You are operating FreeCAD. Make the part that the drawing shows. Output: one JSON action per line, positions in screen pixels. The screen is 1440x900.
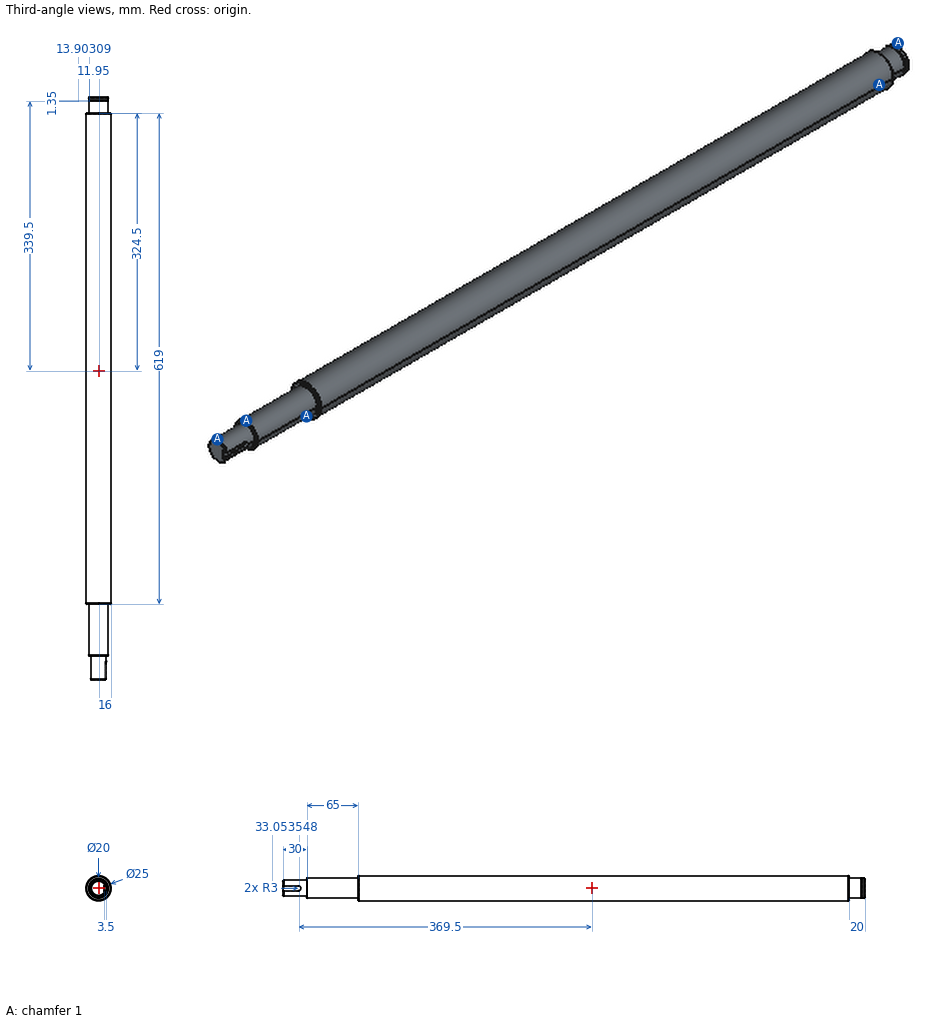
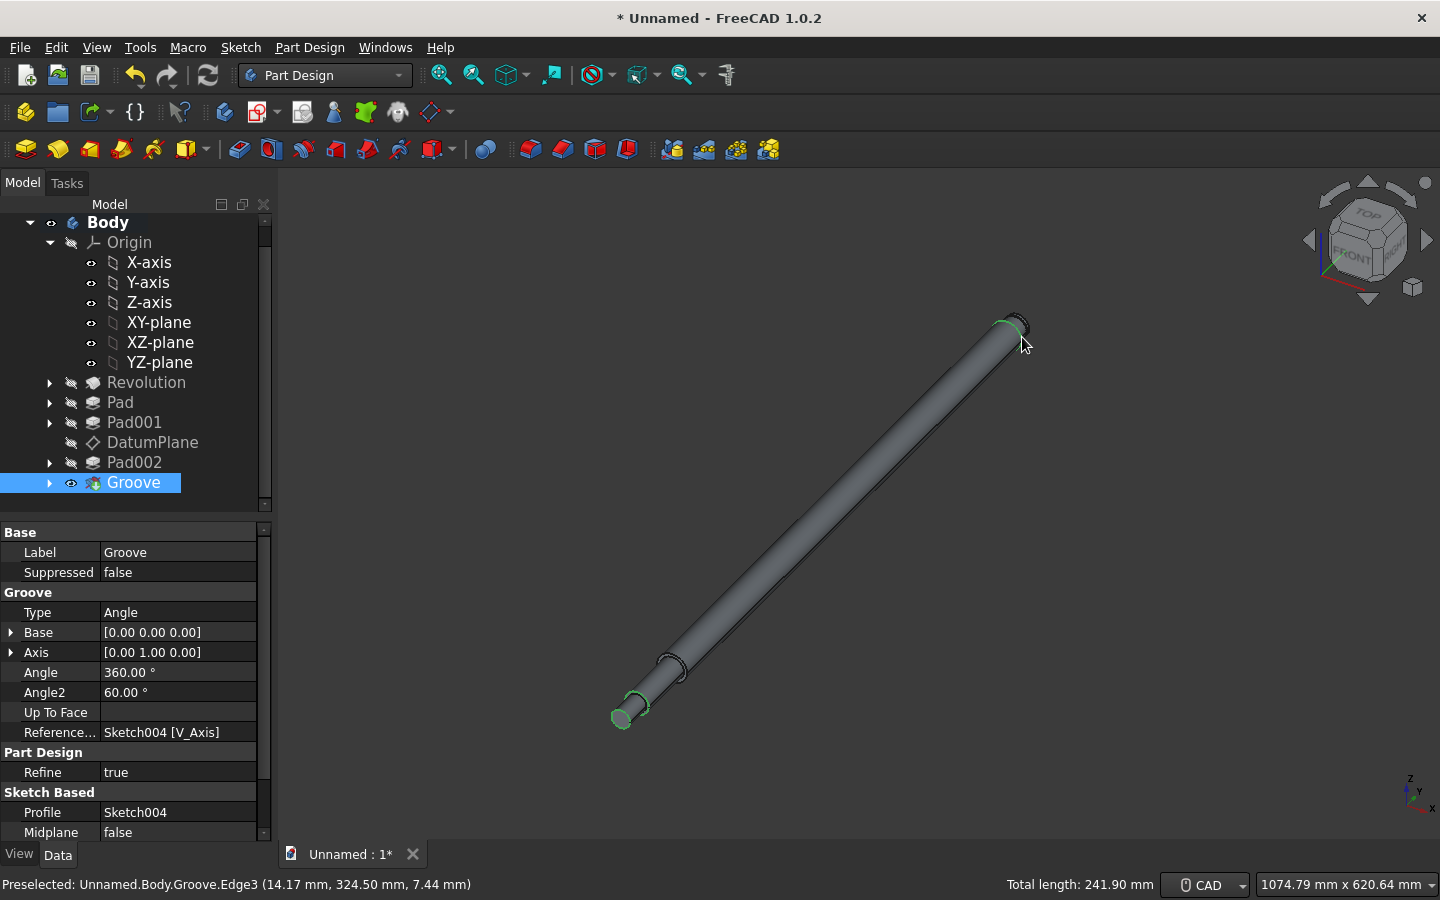
{"action": "left_click", "coordinate": [660, 655], "text": "ctrl"}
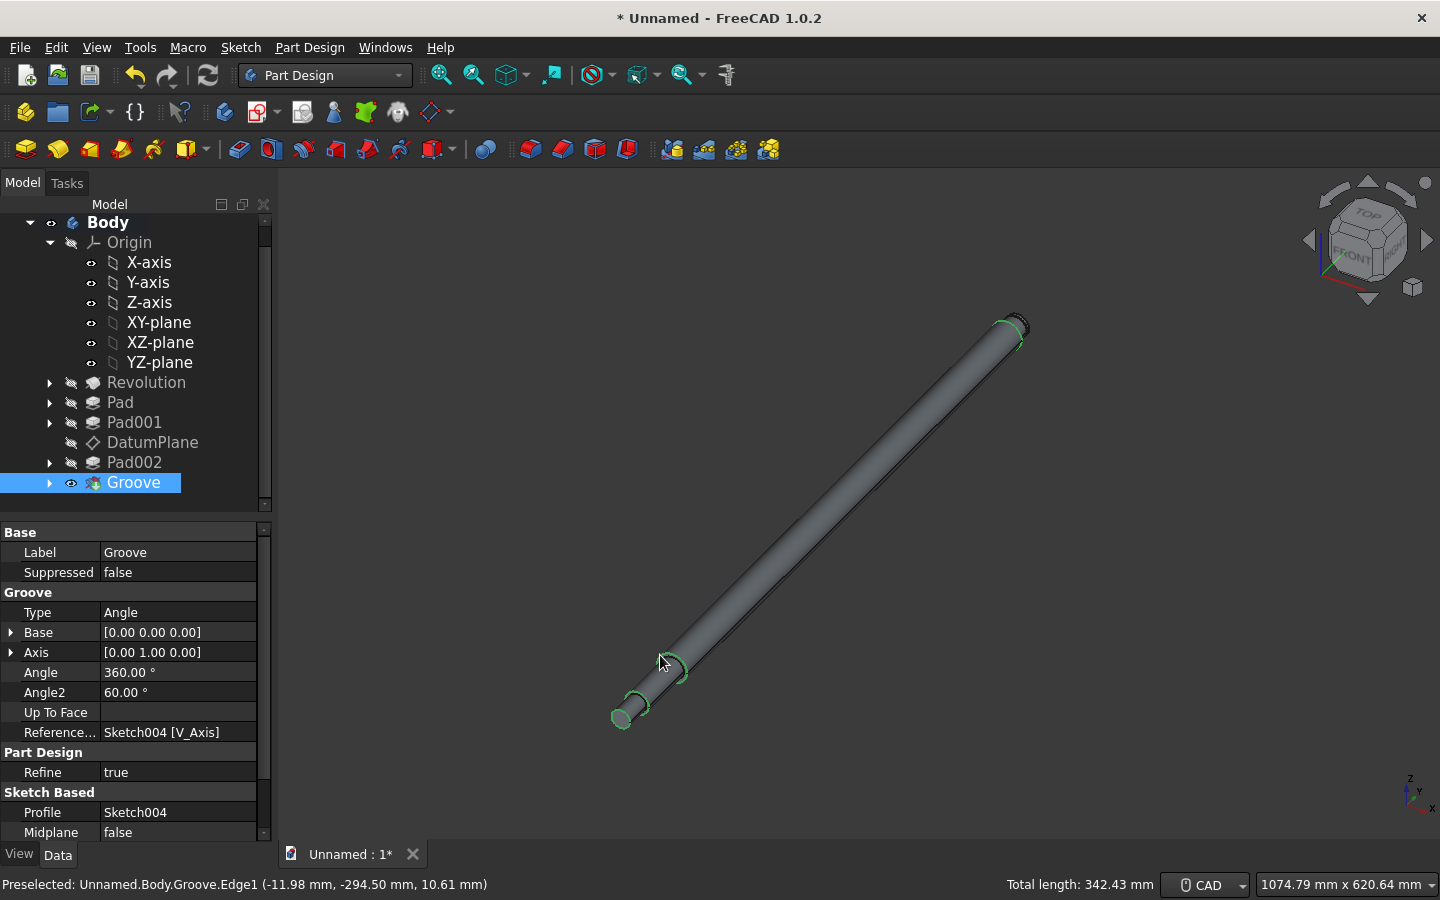
{"action": "key", "text": "0"}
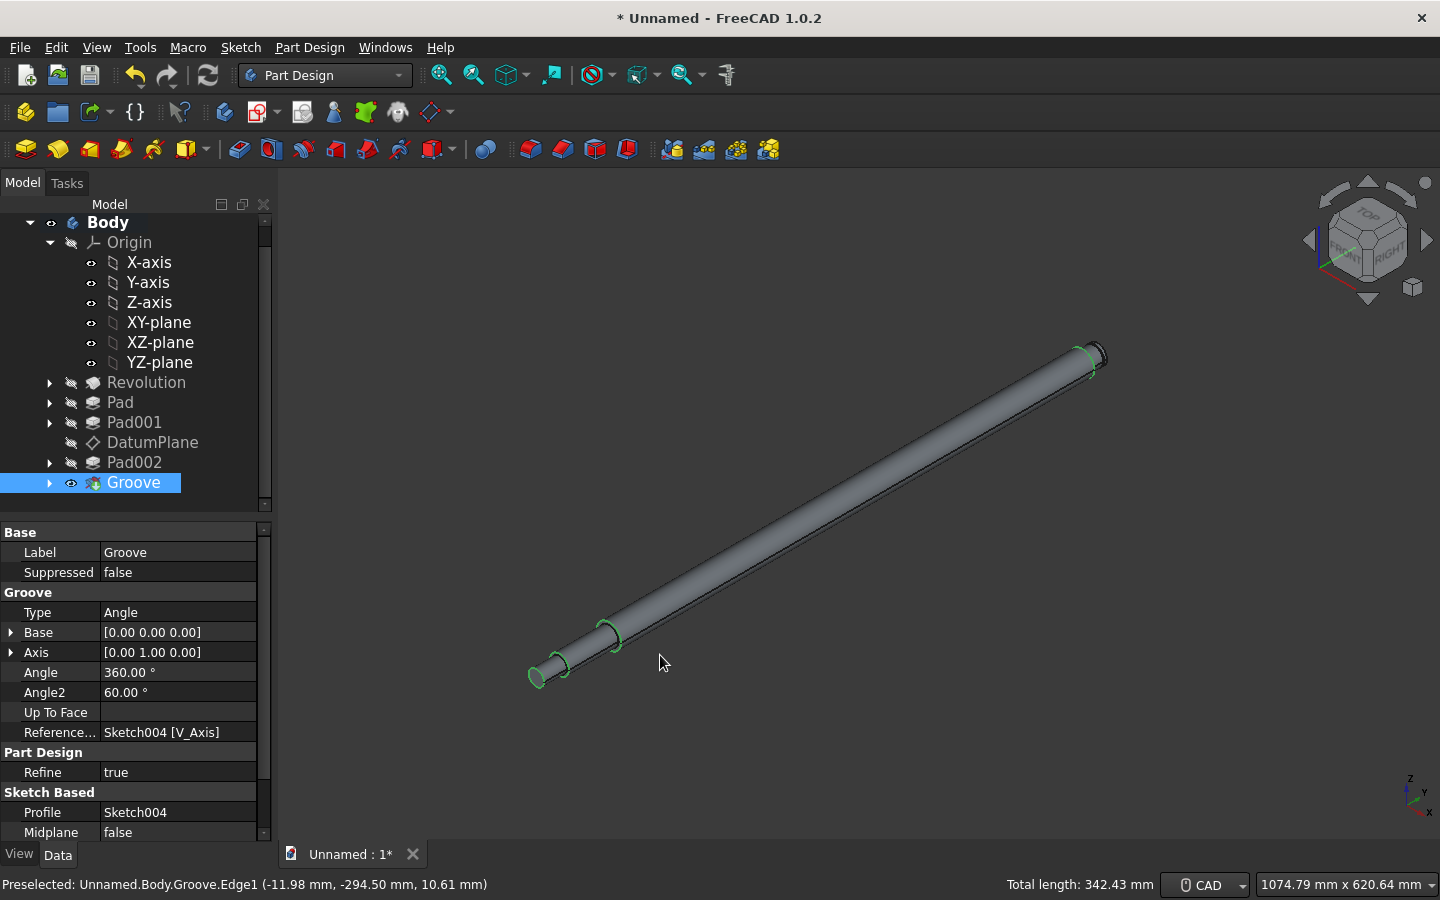
{"action": "key", "text": "2"}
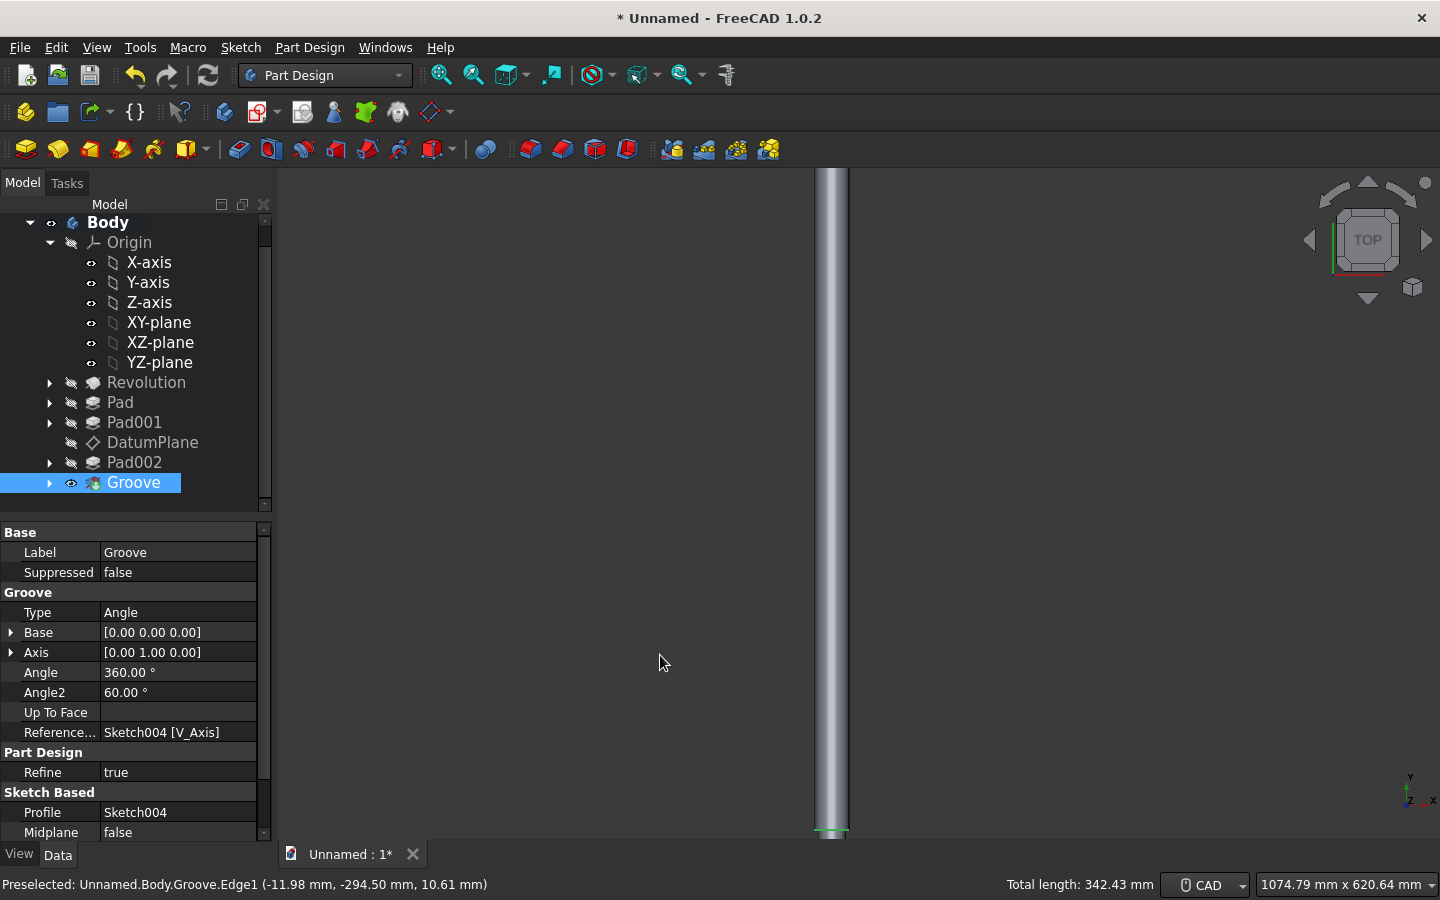
{"action": "left_click", "coordinate": [442, 76]}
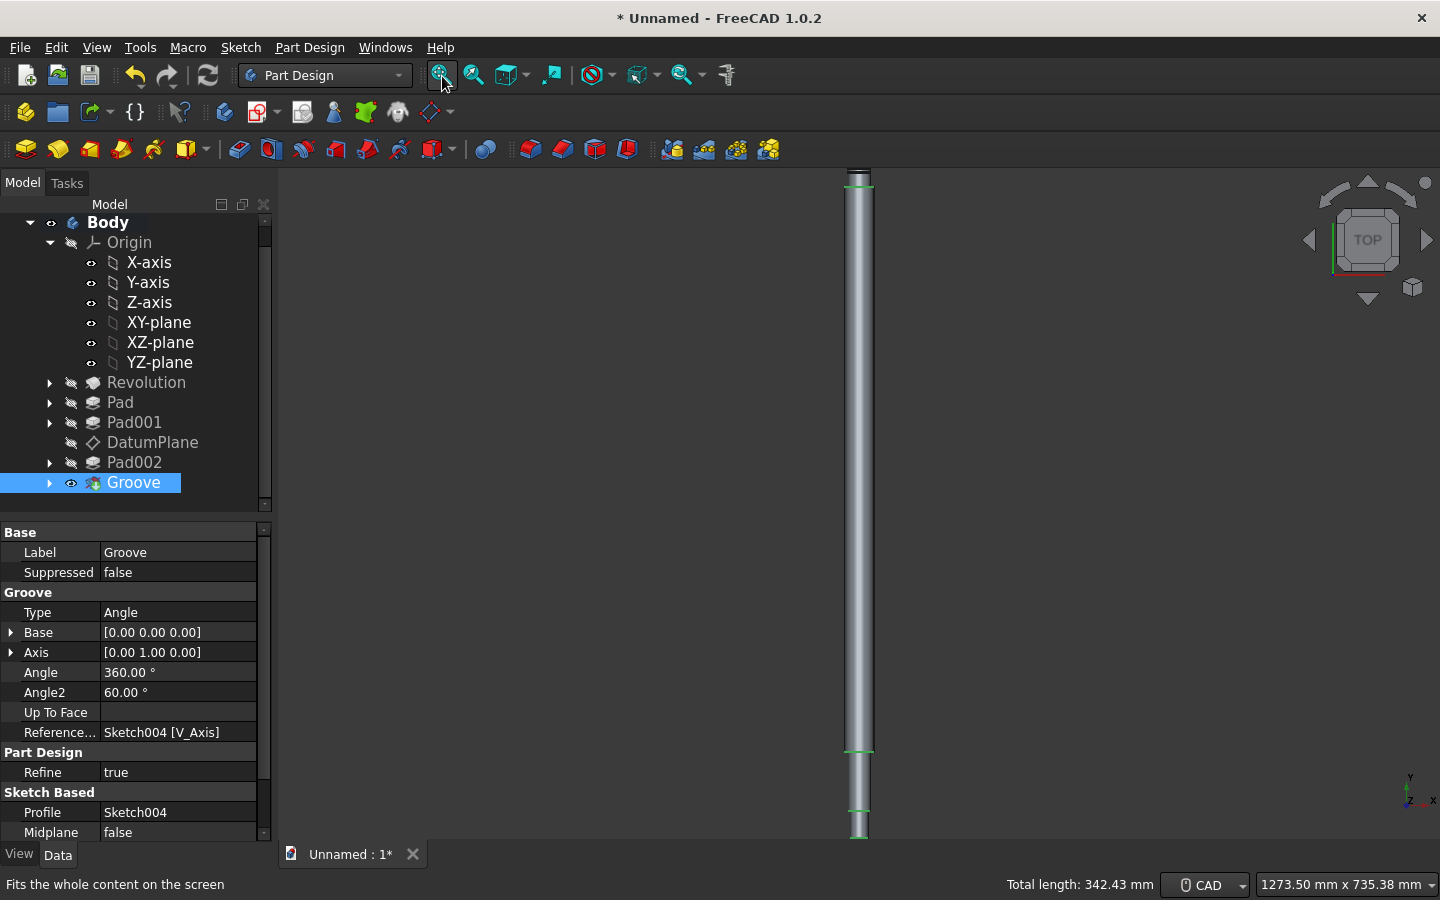
{"action": "key", "text": "1"}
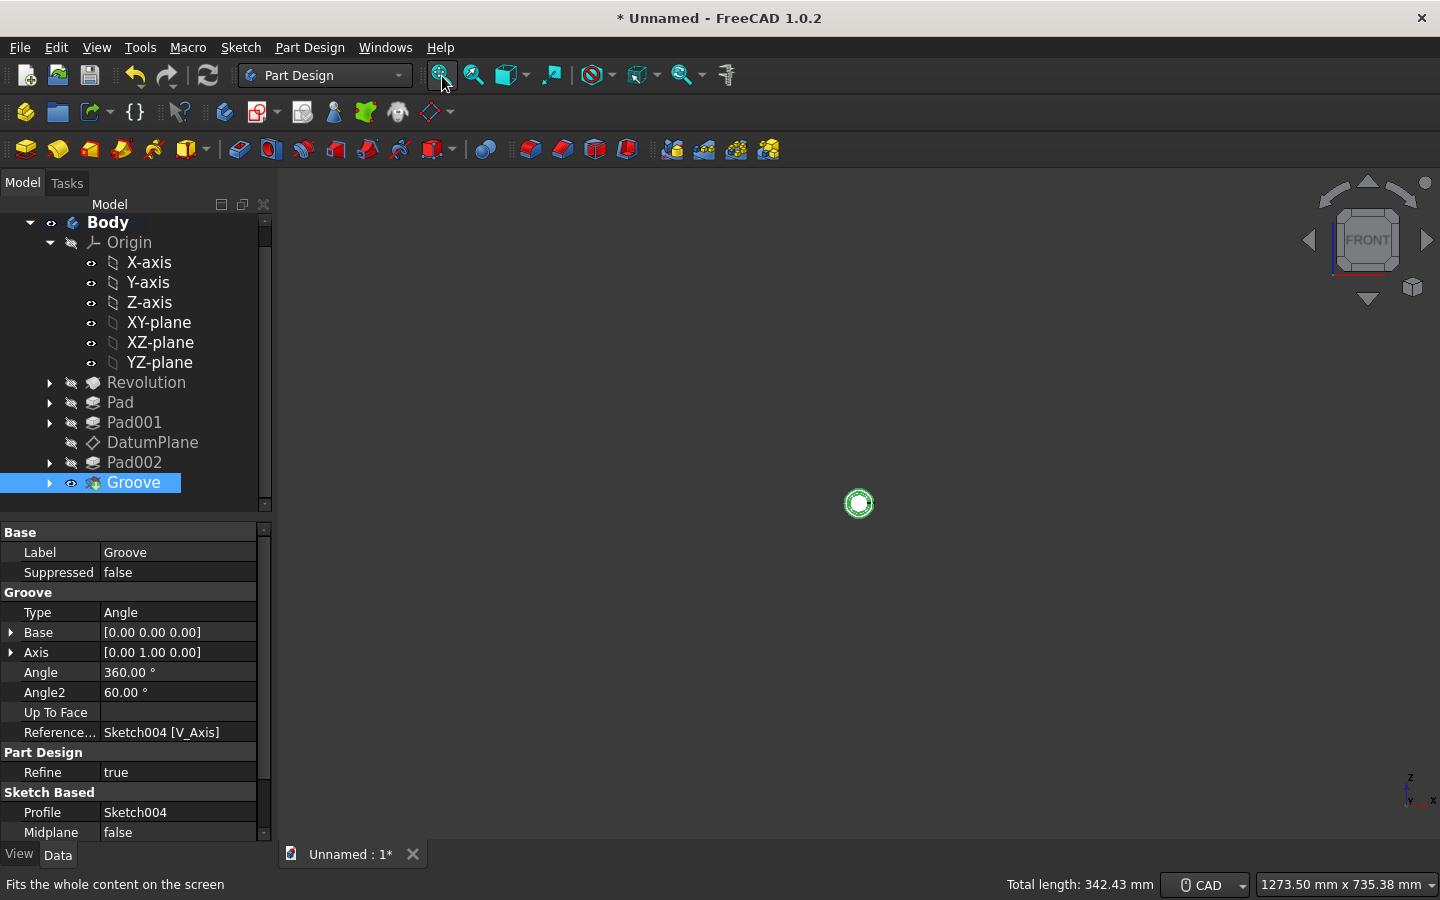
{"action": "left_click", "coordinate": [442, 76]}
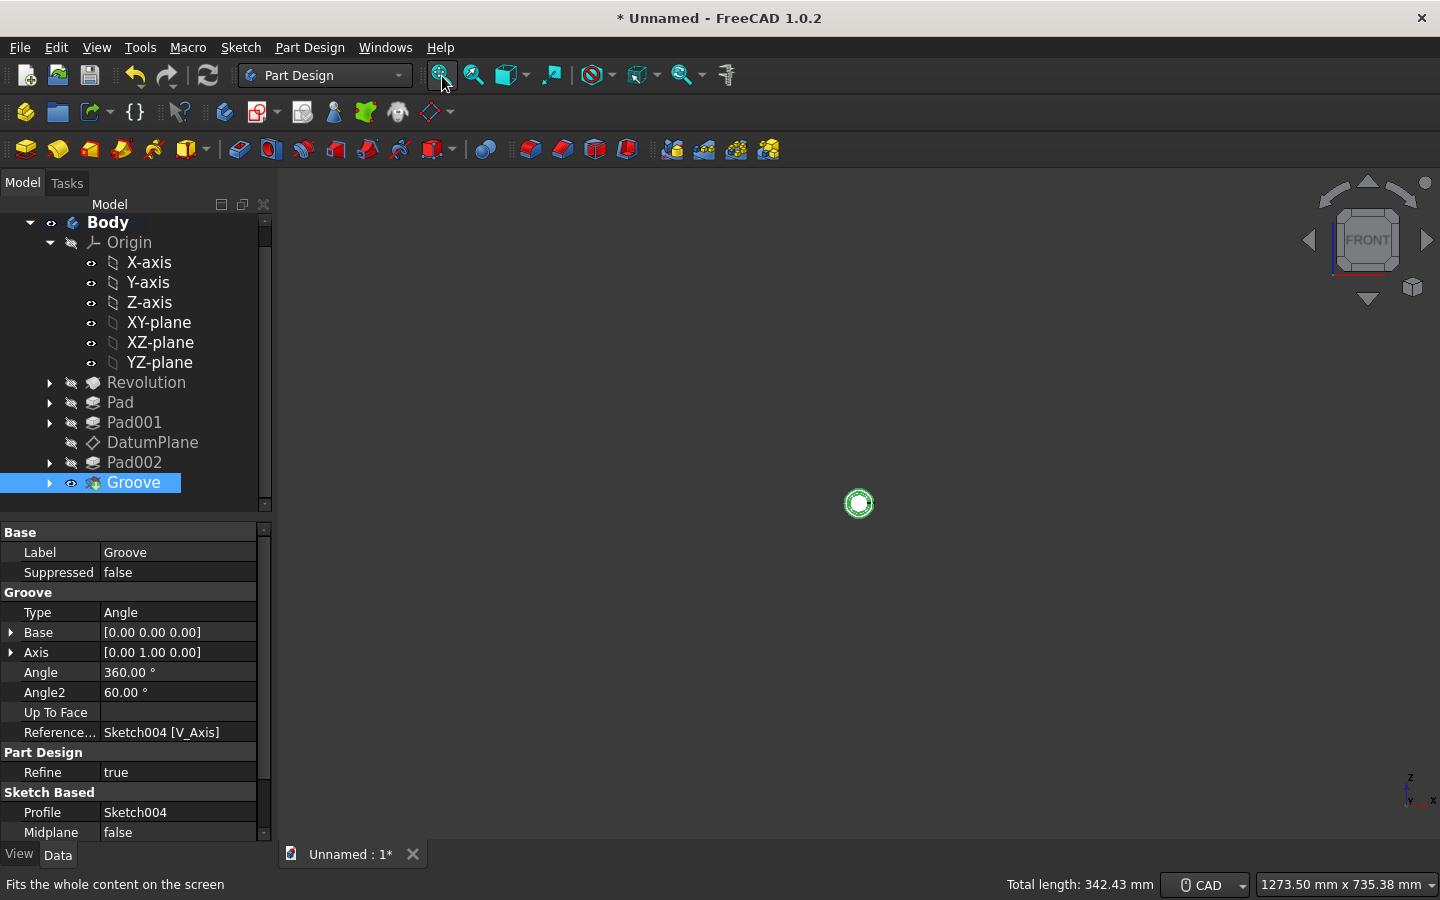
{"action": "key", "text": "3"}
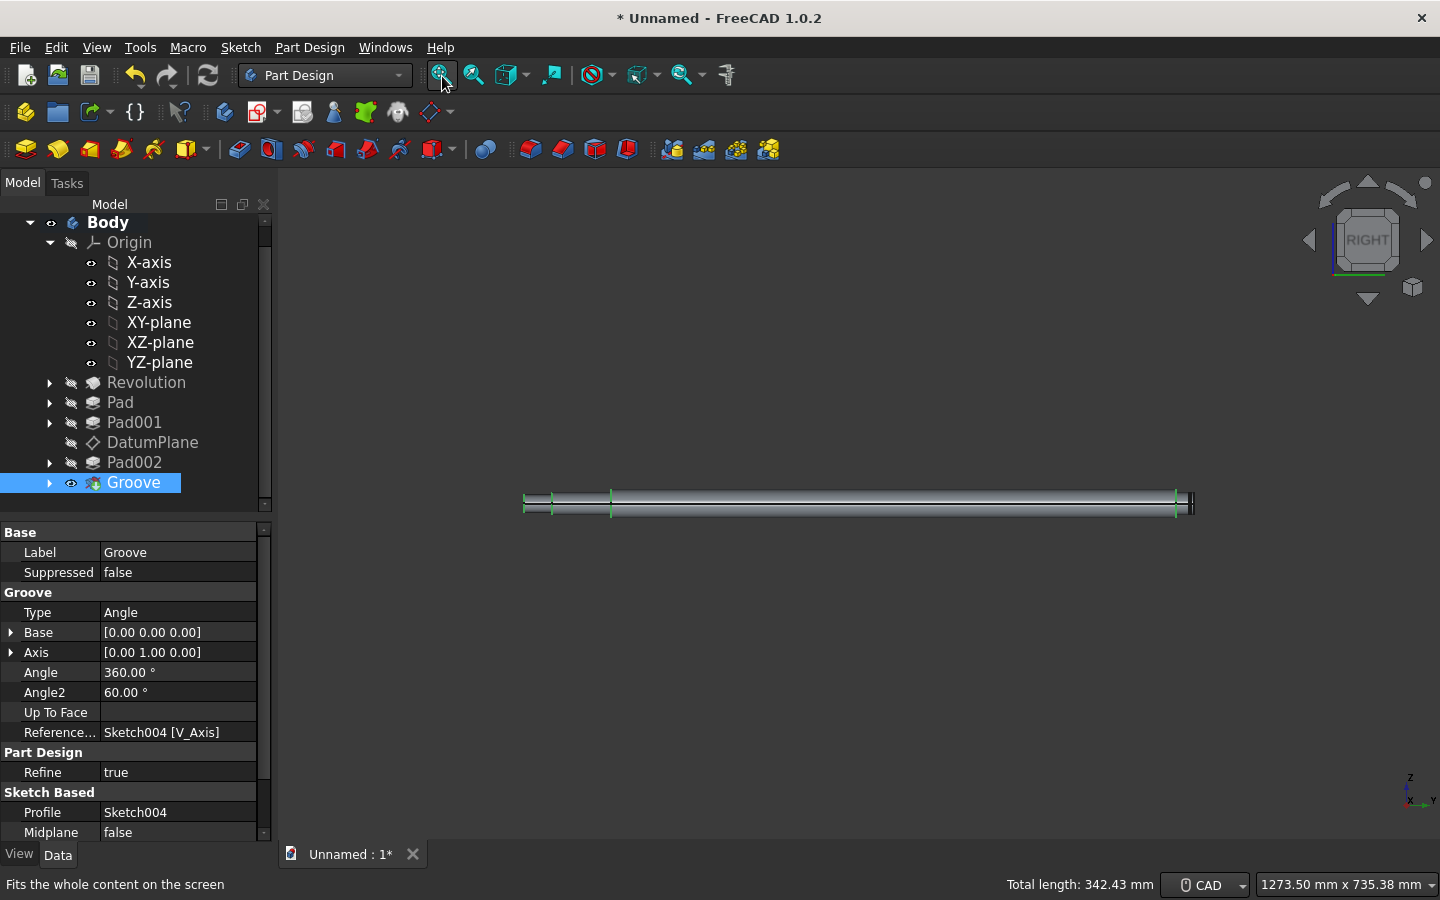
{"action": "key", "text": "5"}